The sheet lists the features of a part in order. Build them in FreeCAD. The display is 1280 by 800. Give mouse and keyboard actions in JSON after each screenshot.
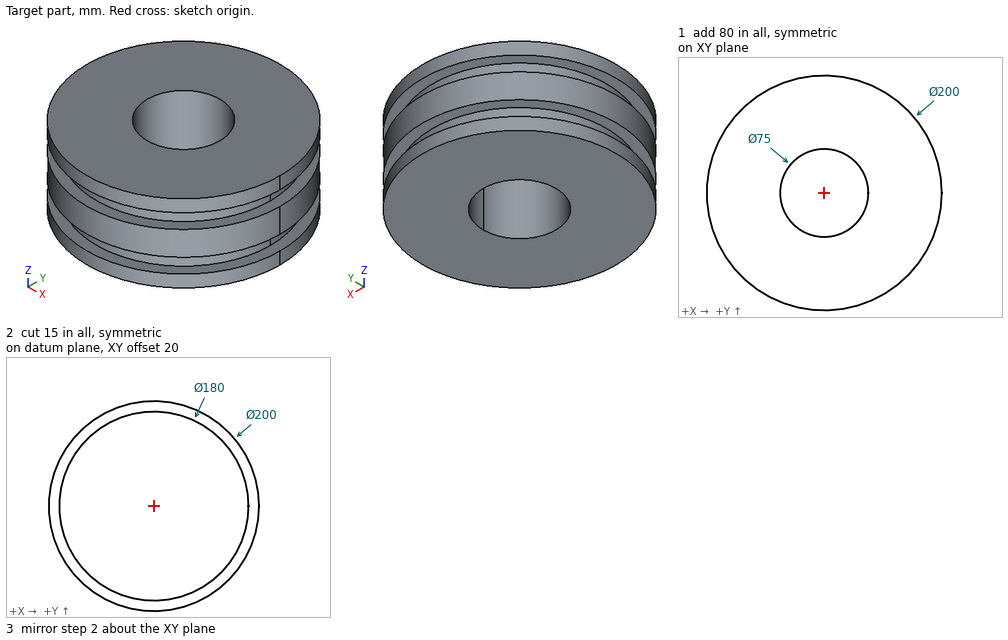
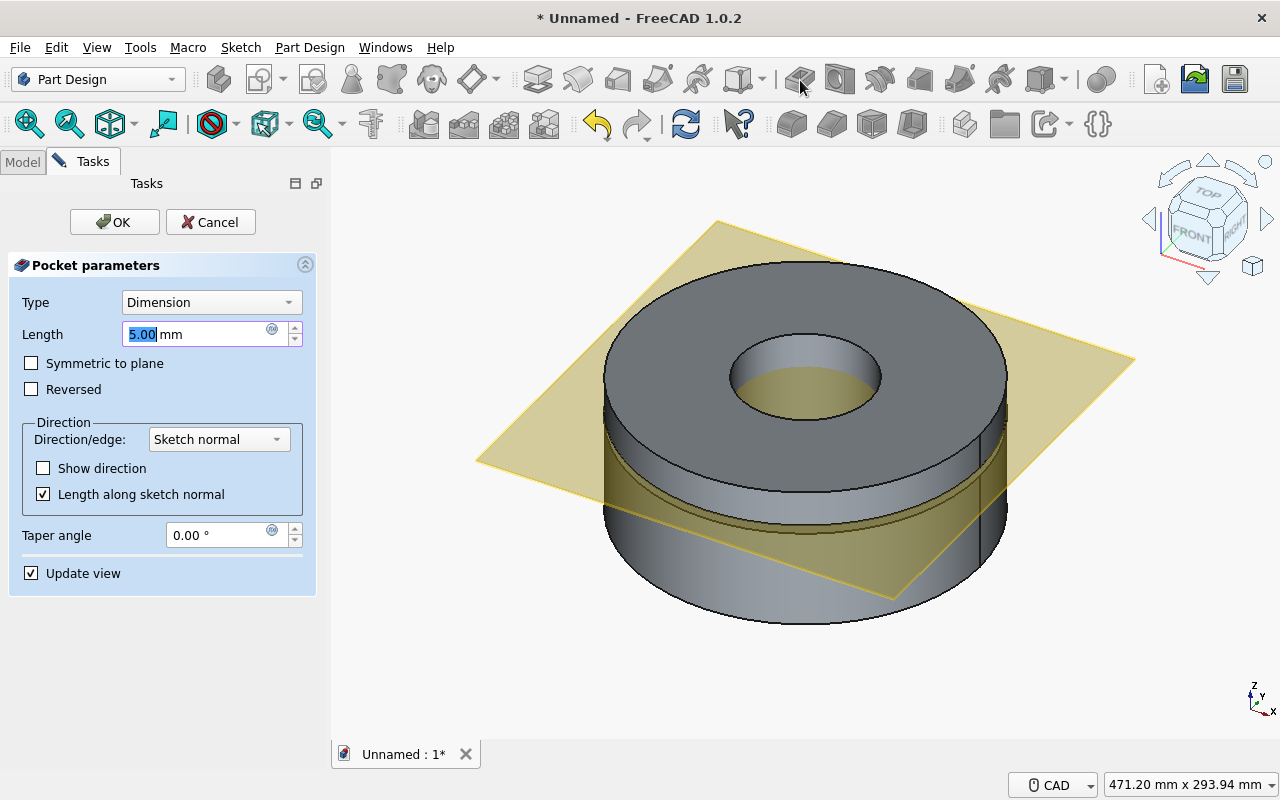
{"action": "type", "text": "15"}
{"action": "key", "text": "Tab"}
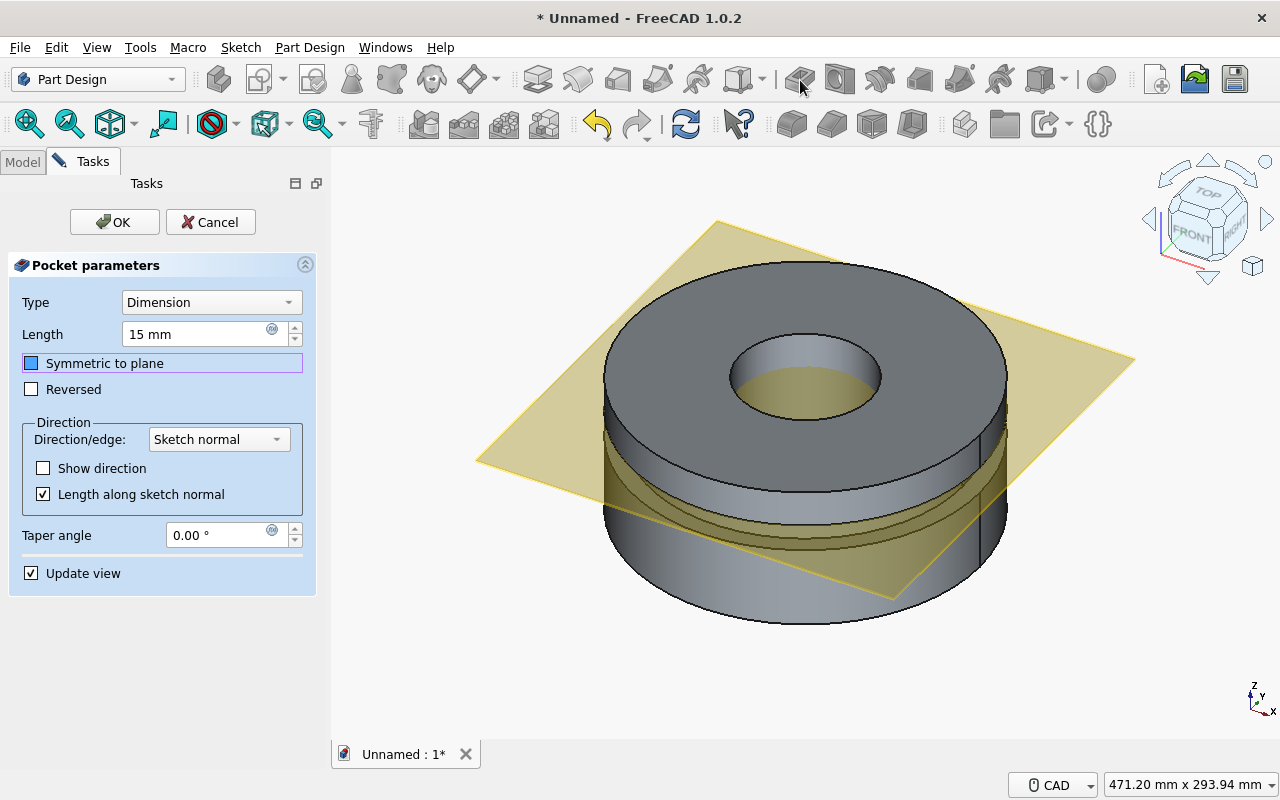
{"action": "left_click", "coordinate": [30, 363]}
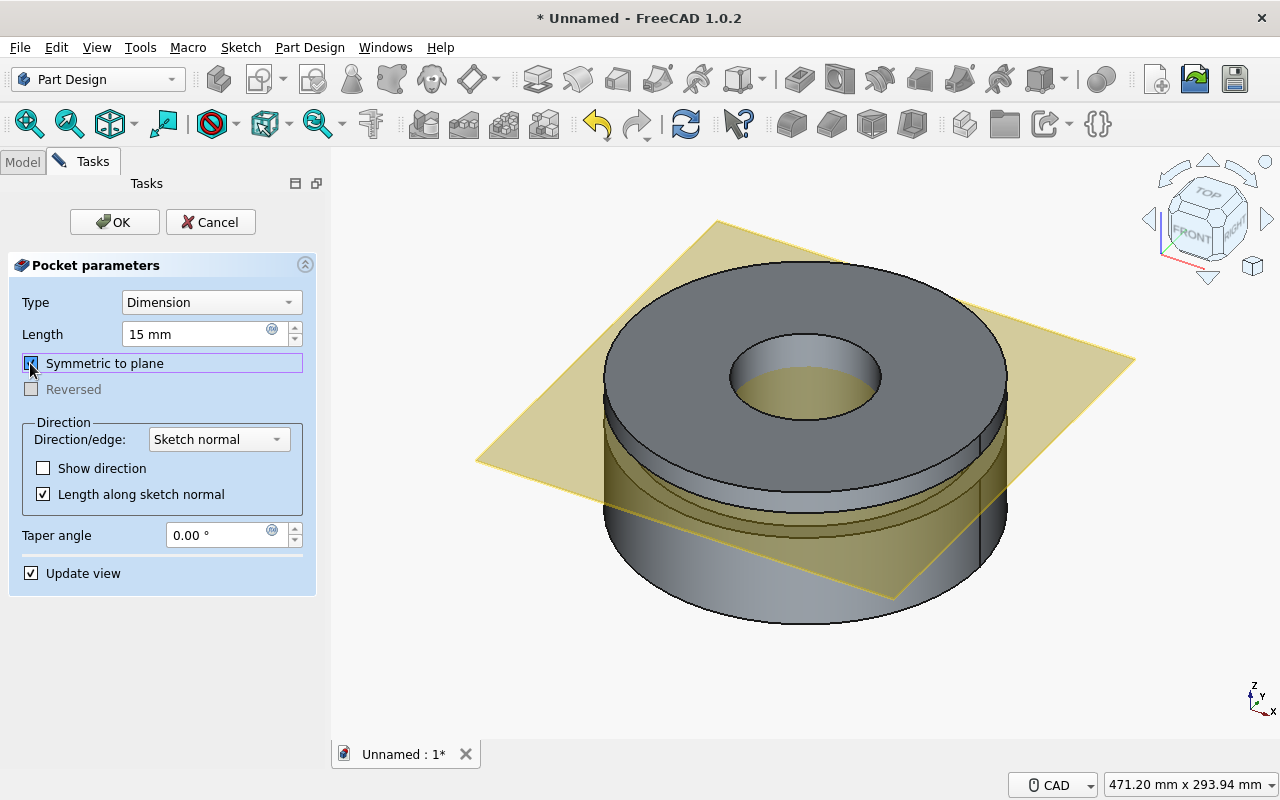
{"action": "left_click", "coordinate": [115, 222]}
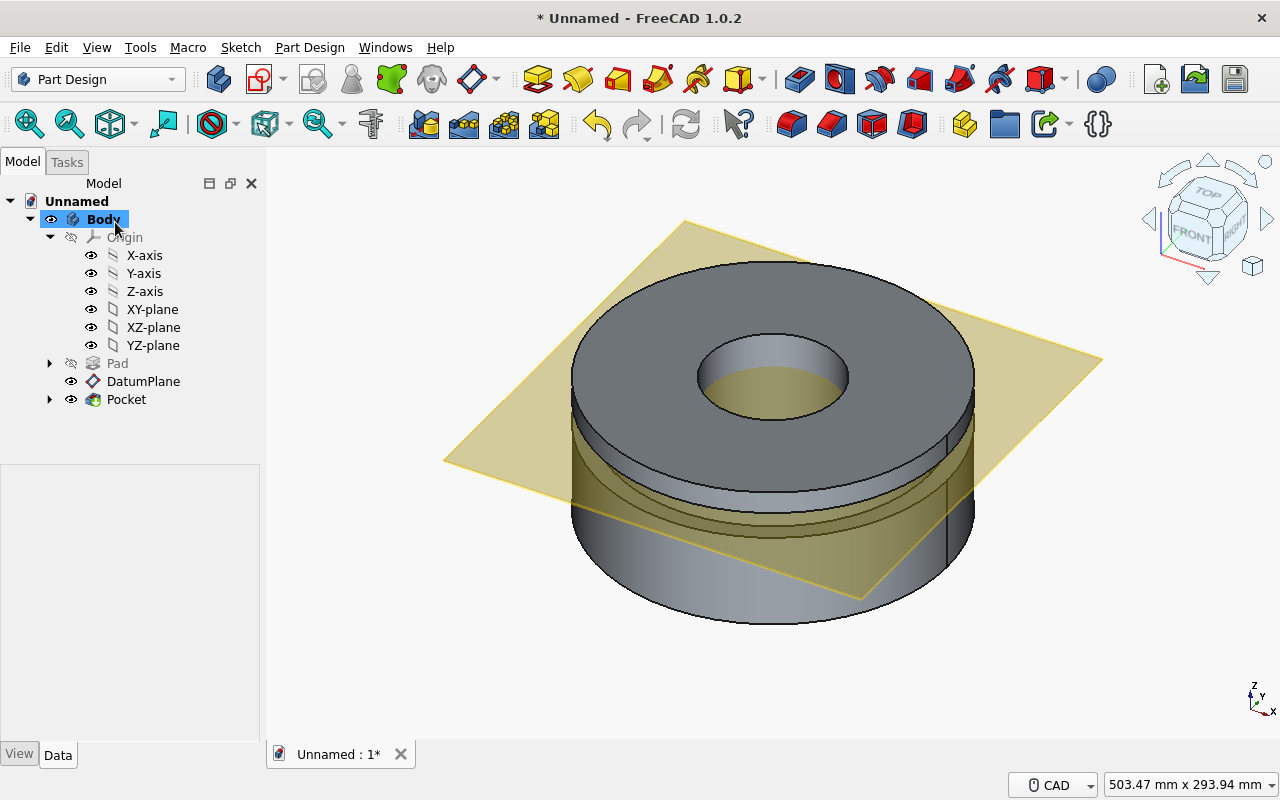
{"action": "left_click", "coordinate": [116, 381]}
{"action": "key", "text": "space"}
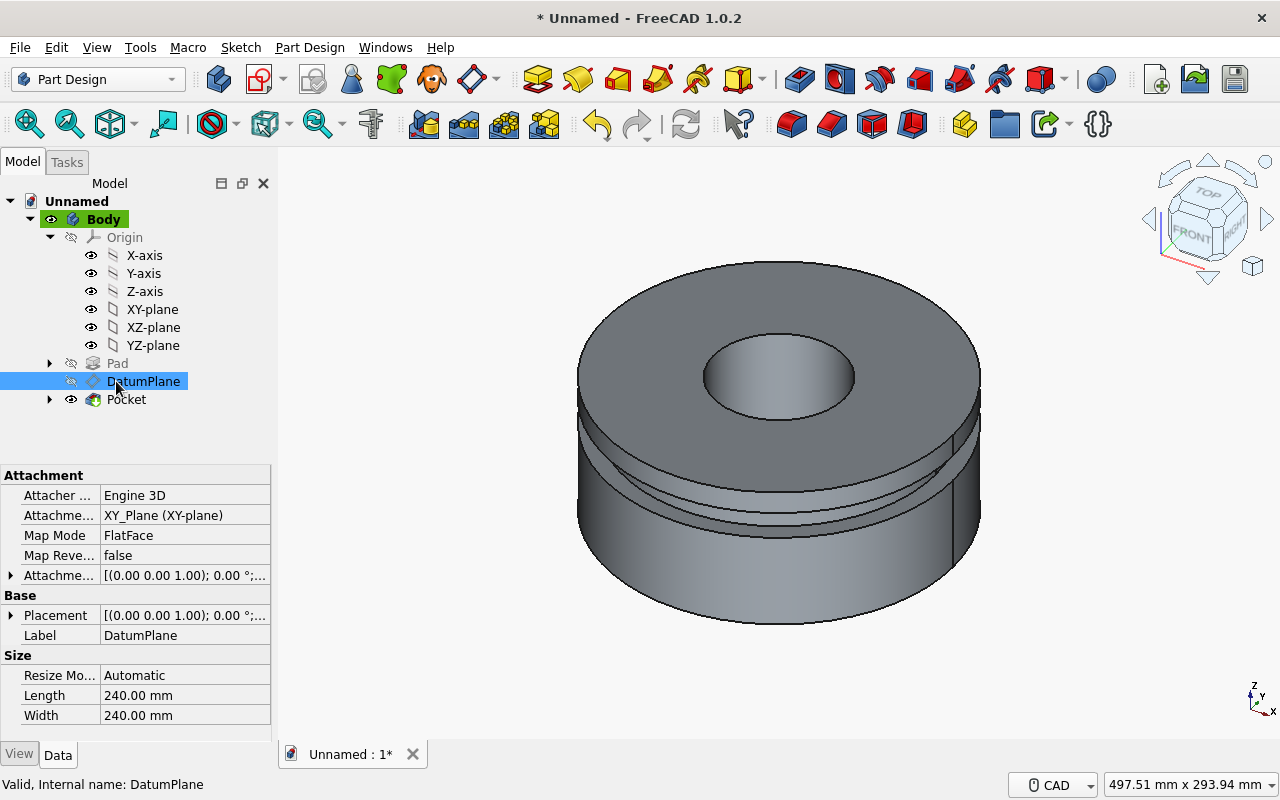
{"action": "left_click", "coordinate": [116, 399]}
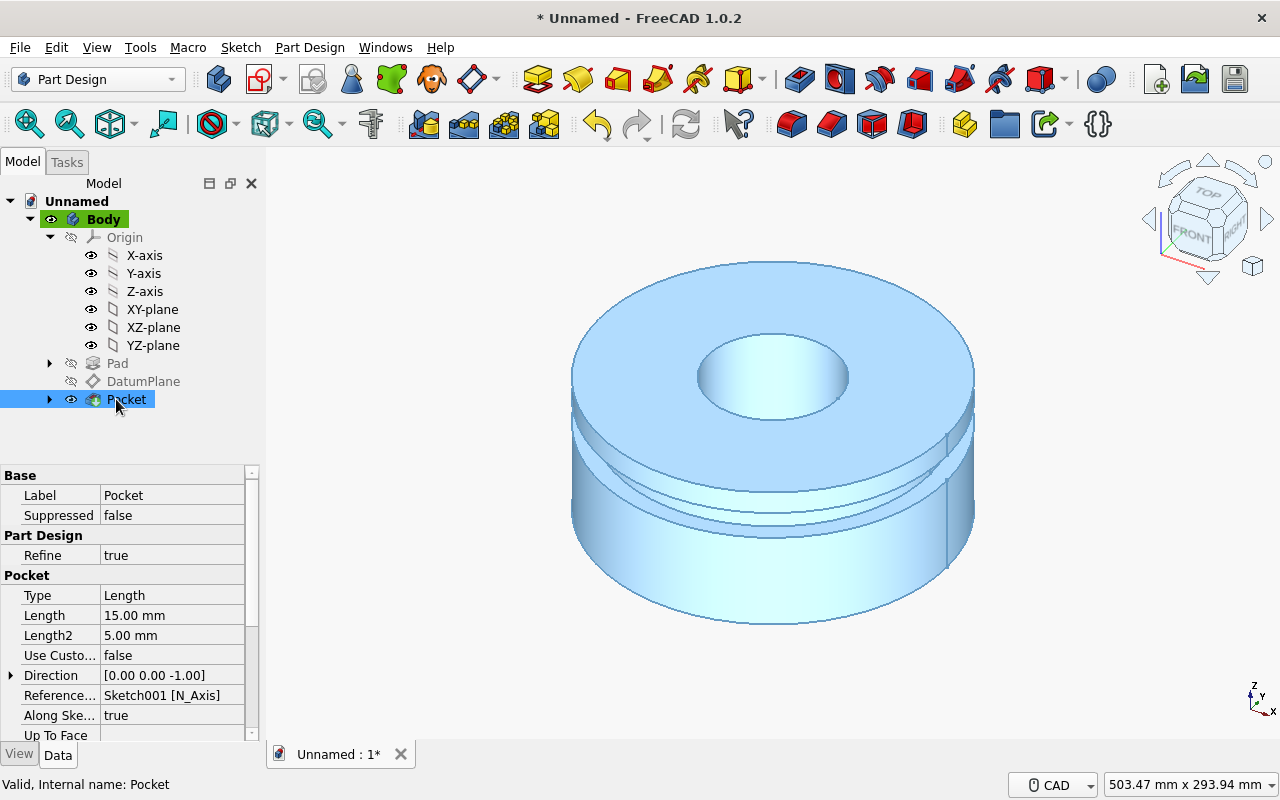
{"action": "left_click", "coordinate": [424, 124]}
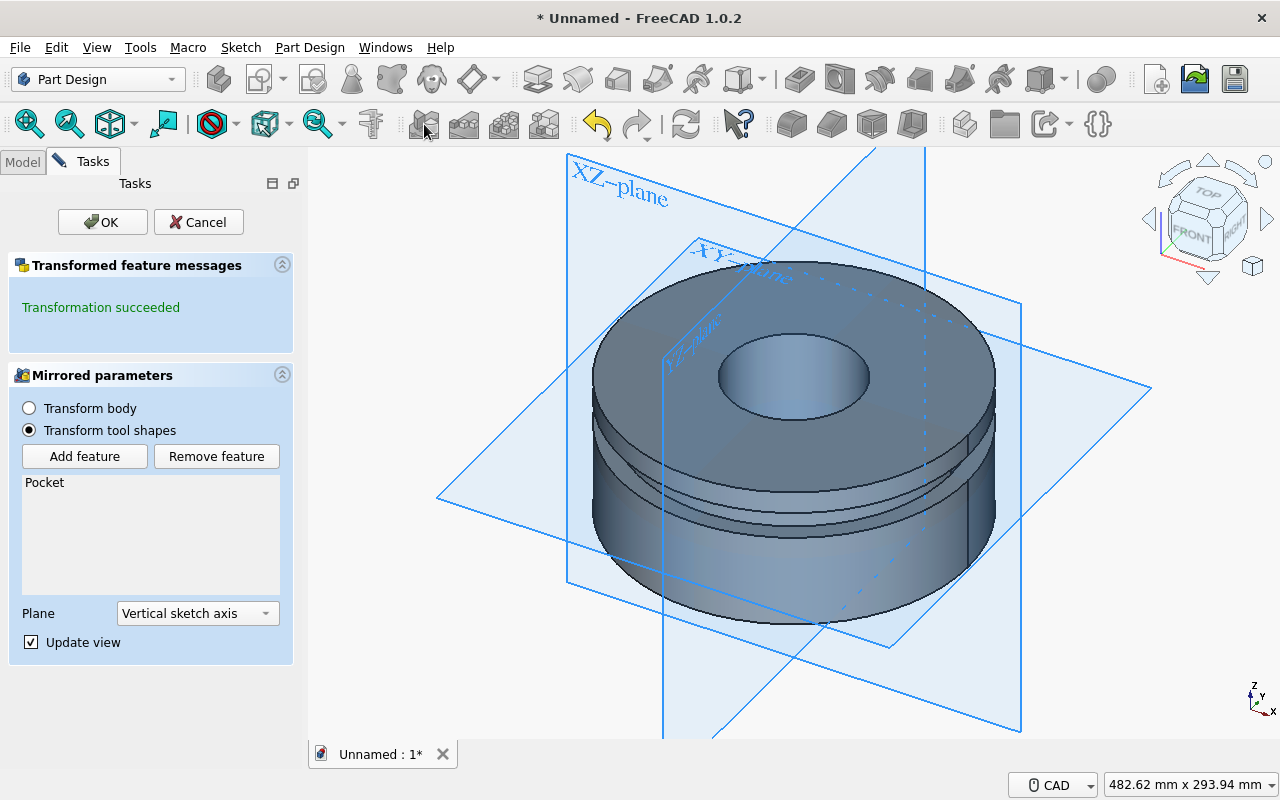
{"action": "left_click", "coordinate": [198, 614]}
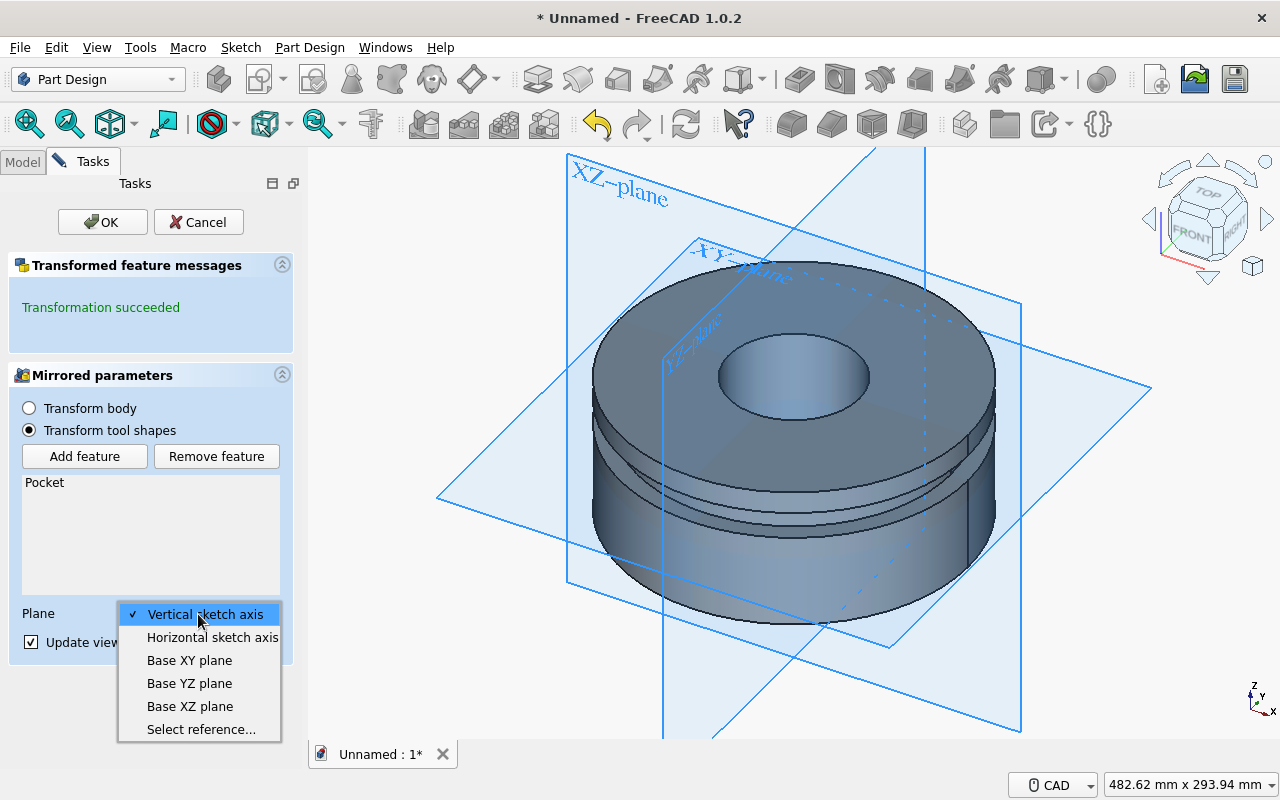
{"action": "left_click", "coordinate": [198, 660]}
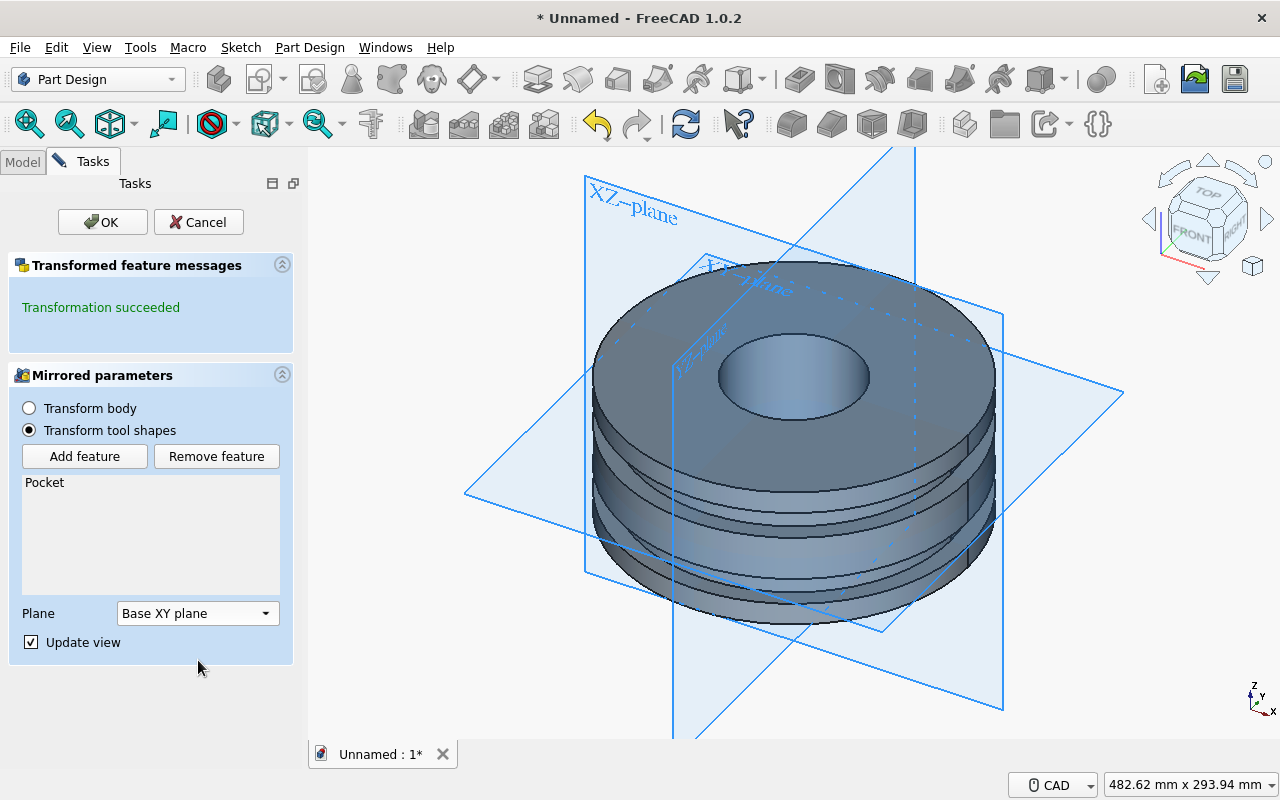
{"action": "left_click", "coordinate": [103, 222]}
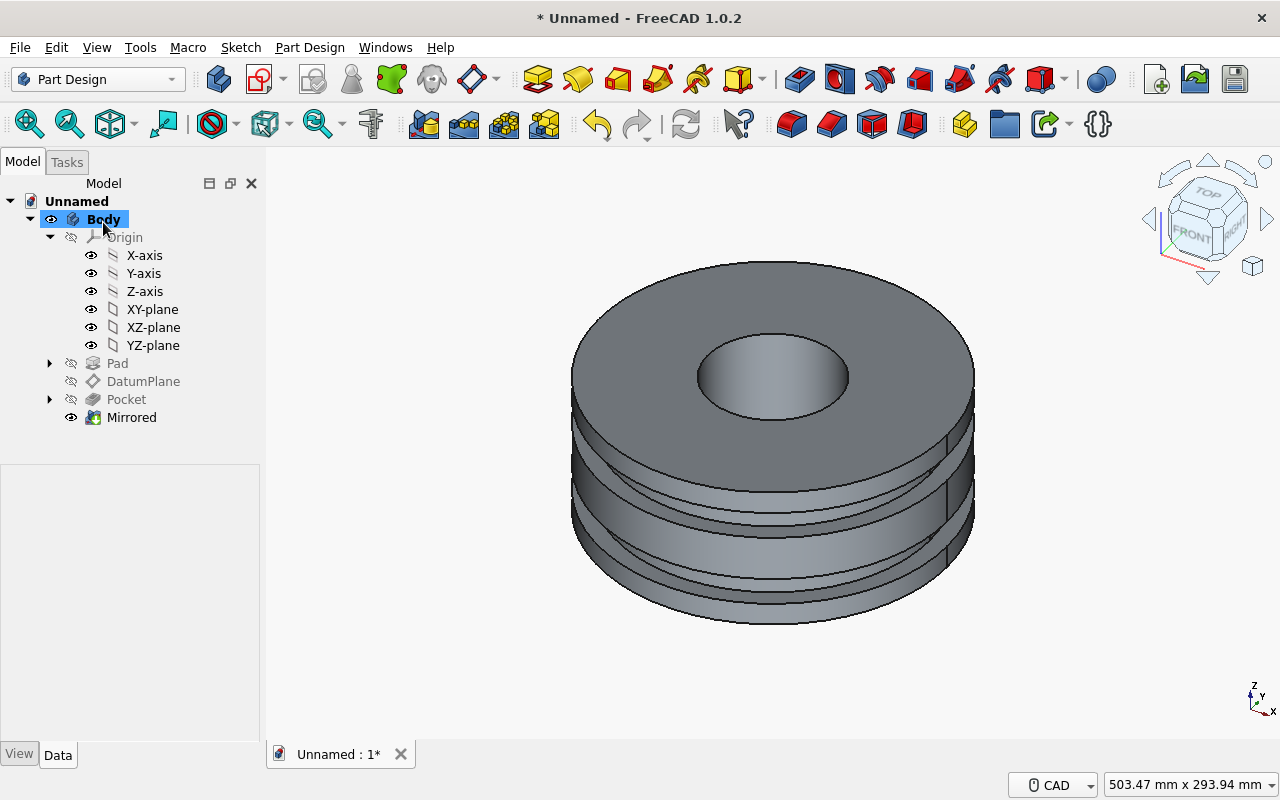
{"action": "key", "text": "0"}